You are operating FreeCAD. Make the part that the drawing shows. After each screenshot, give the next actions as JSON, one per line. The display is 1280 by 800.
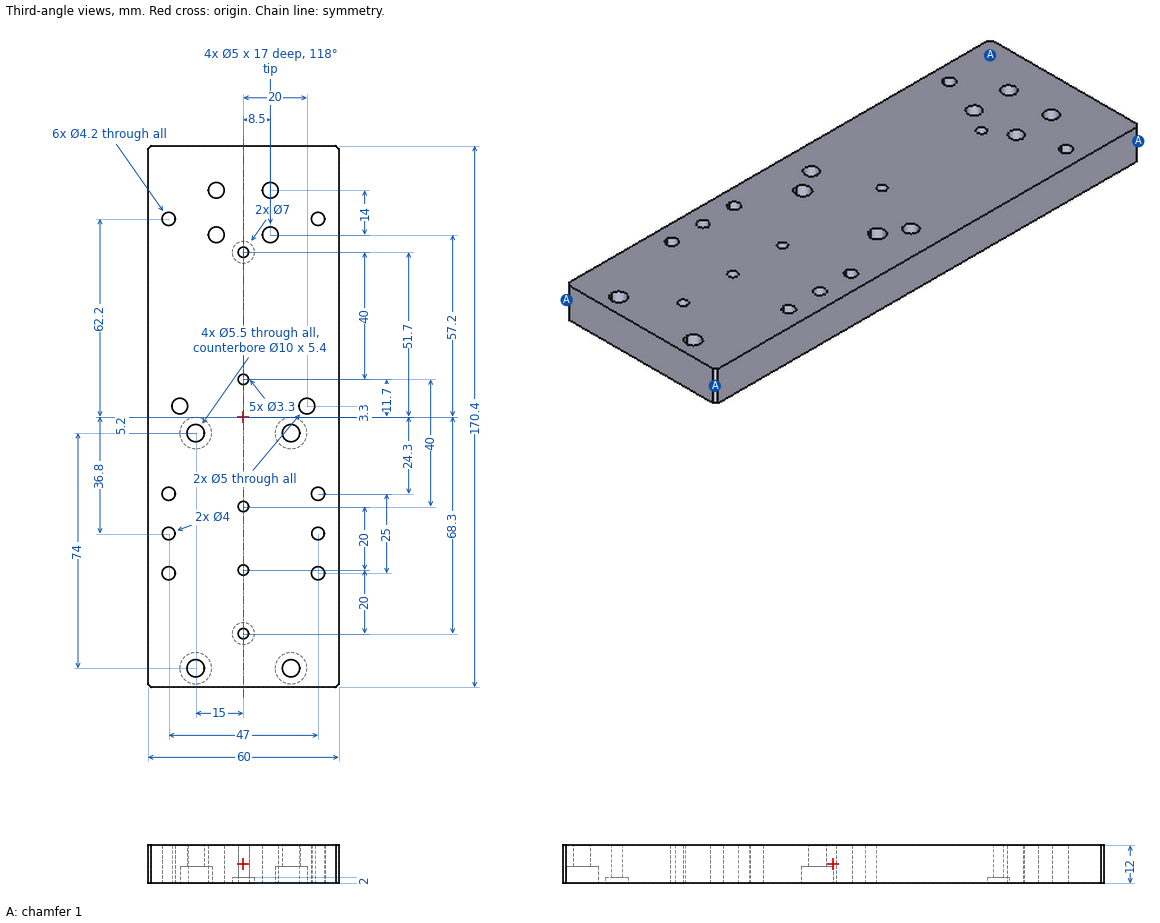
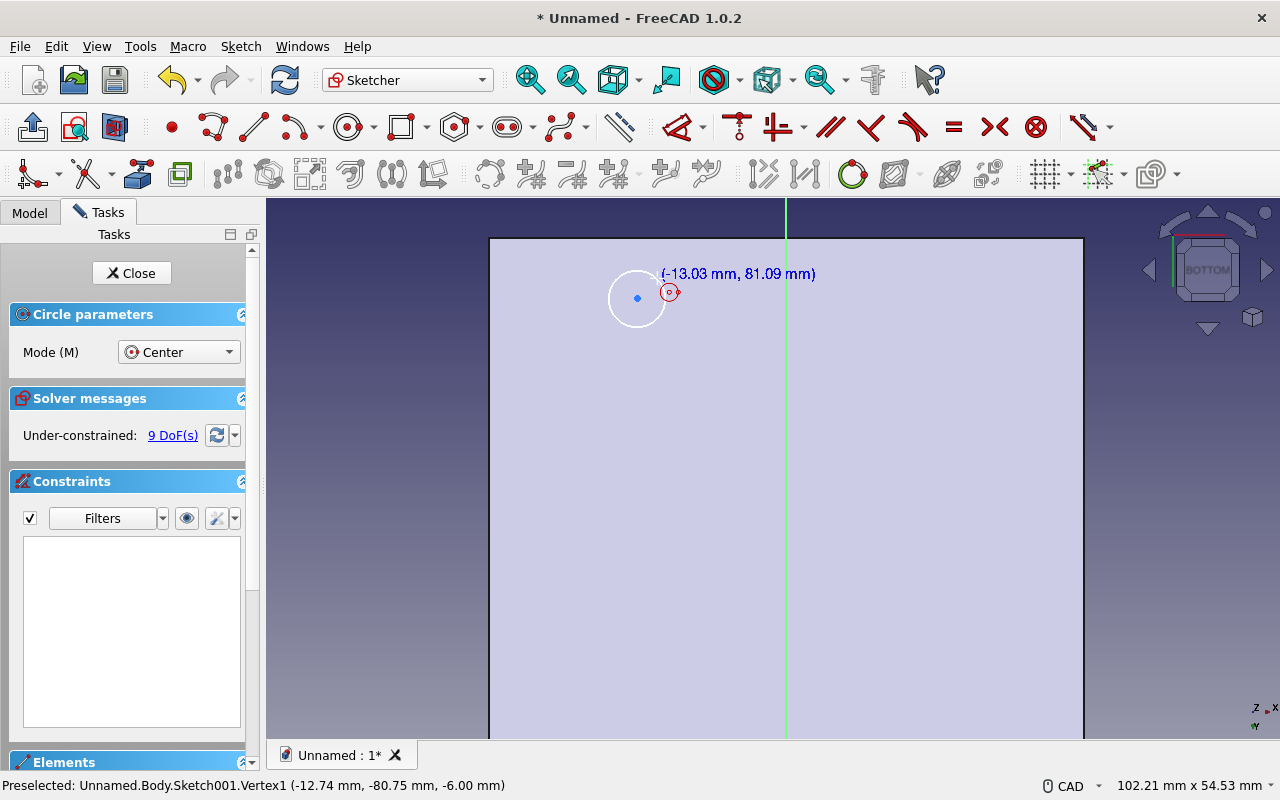
{"action": "left_click", "coordinate": [935, 298]}
{"action": "left_click", "coordinate": [954, 278]}
{"action": "key", "text": "Escape"}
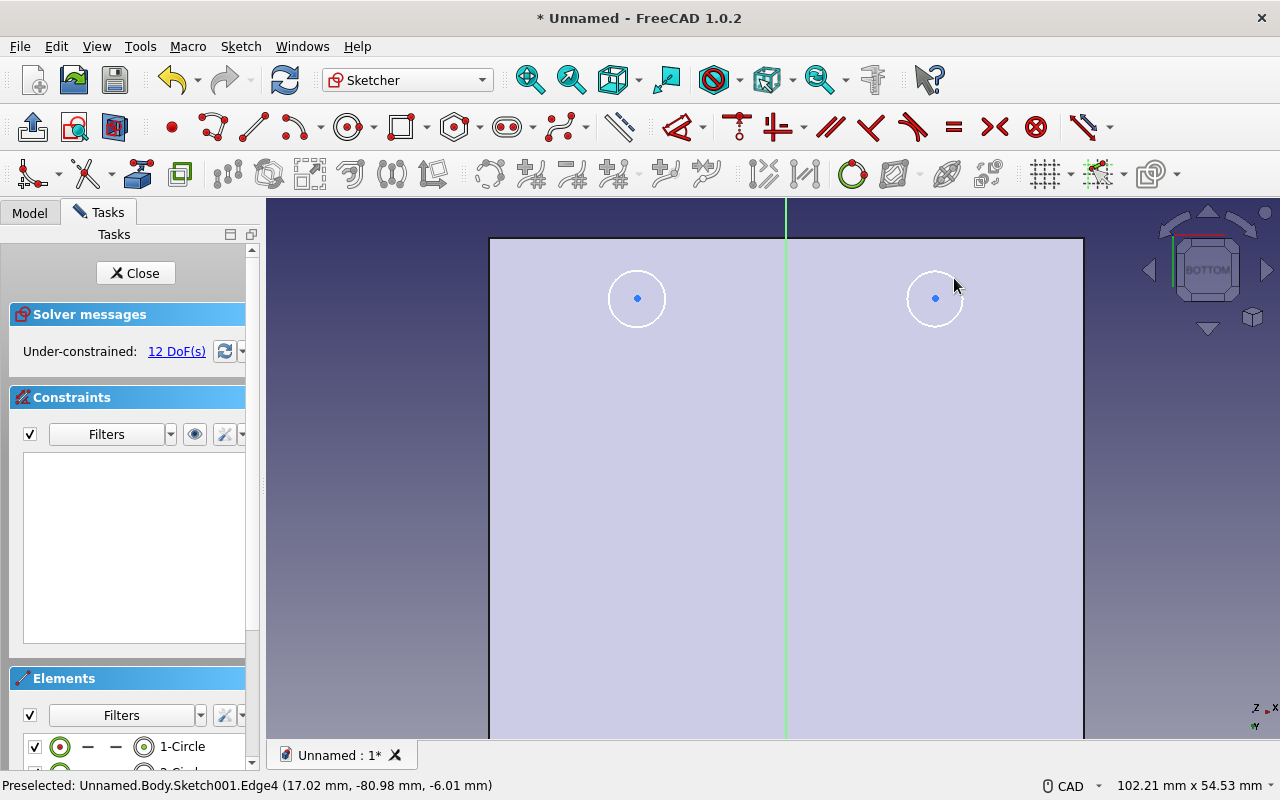
{"action": "scroll", "coordinate": [638, 298], "scroll_direction": "down", "scroll_amount": 4}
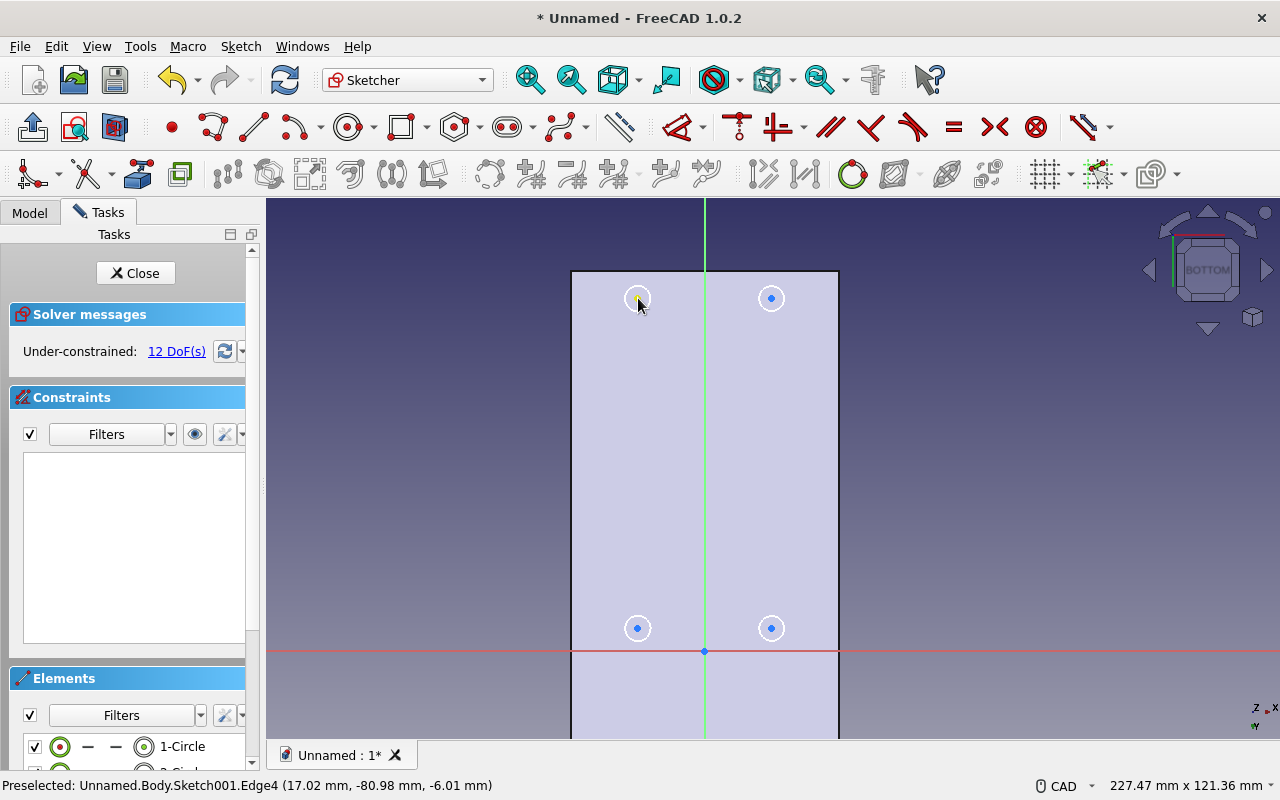
{"action": "left_click", "coordinate": [647, 619]}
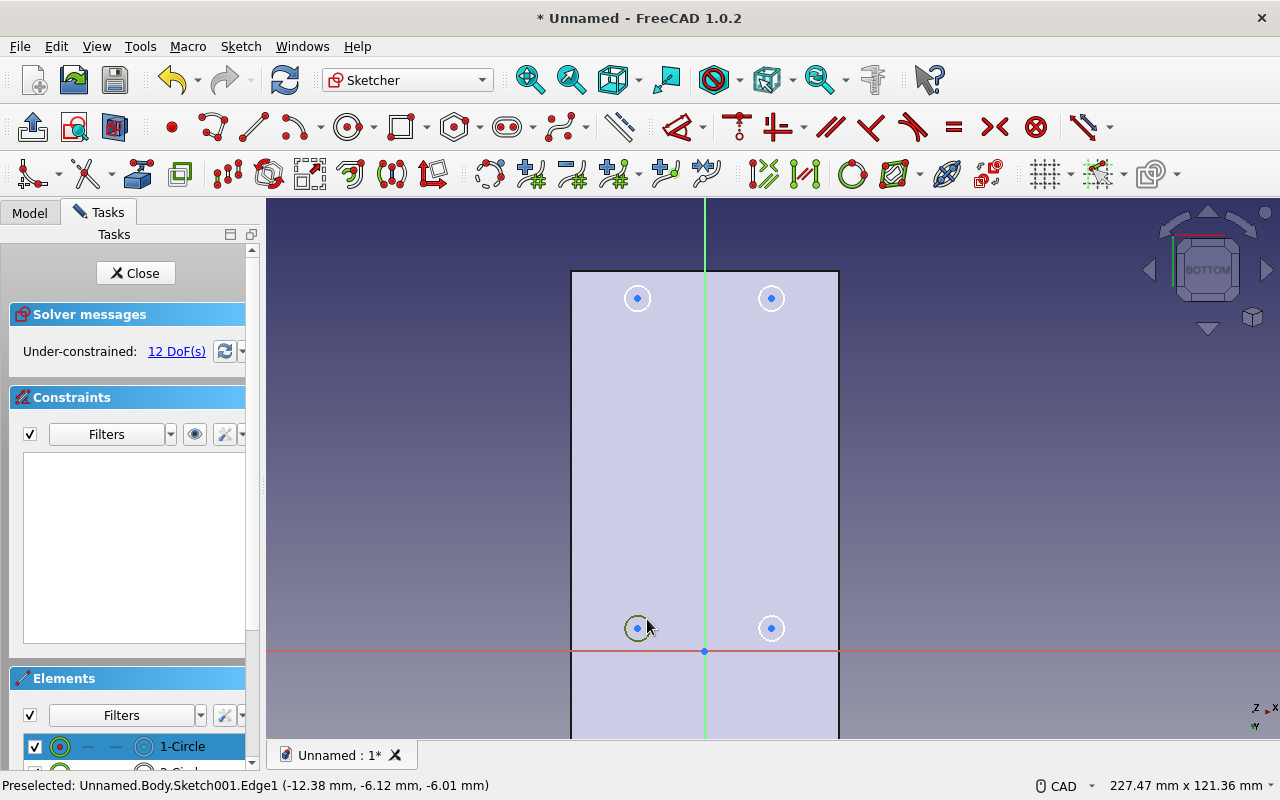
{"action": "left_click", "coordinate": [780, 620]}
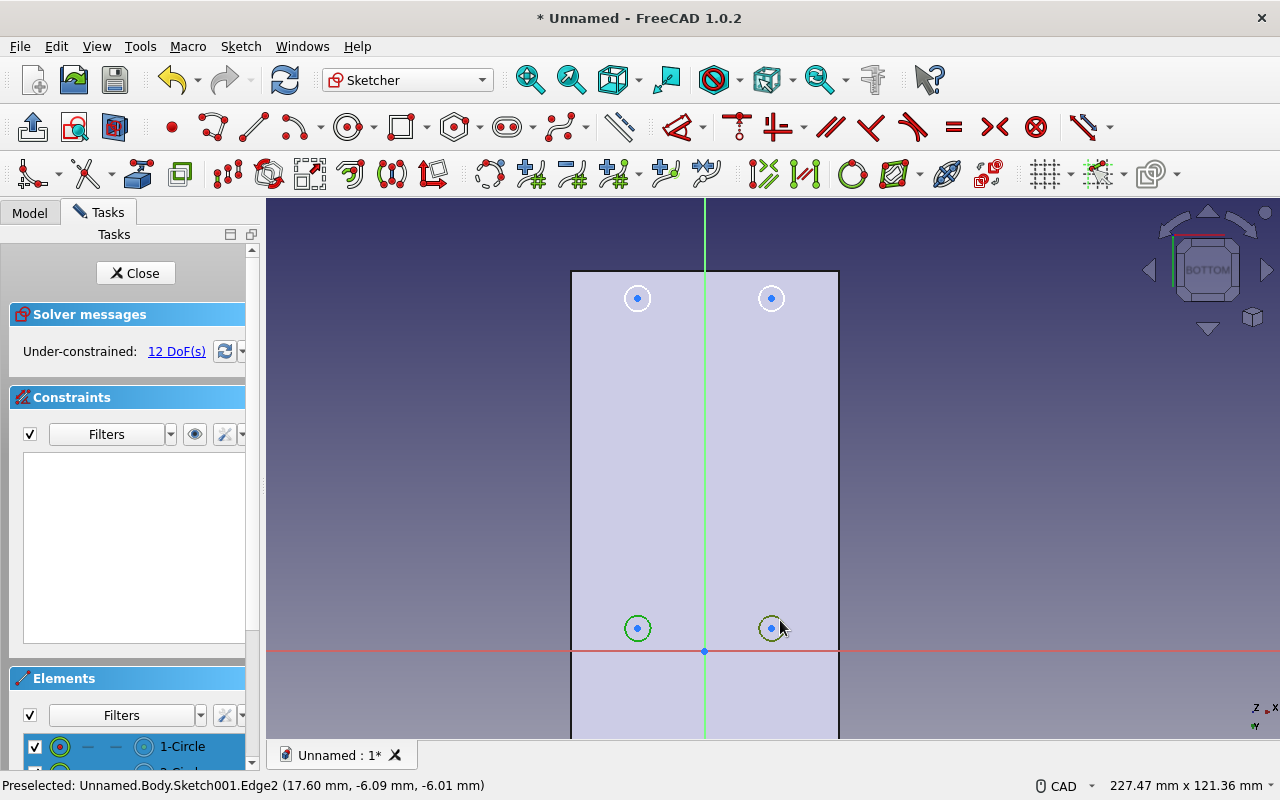
{"action": "left_click", "coordinate": [647, 290]}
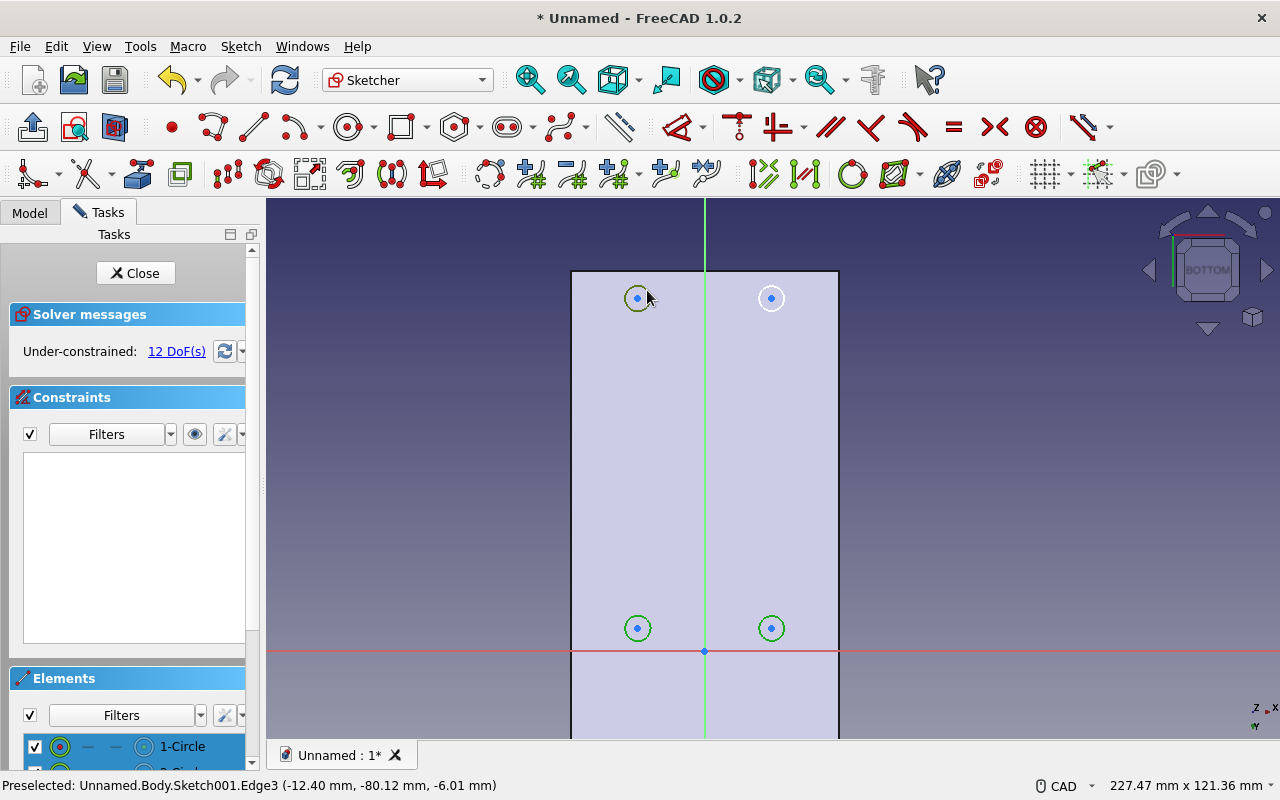
{"action": "left_click", "coordinate": [780, 290]}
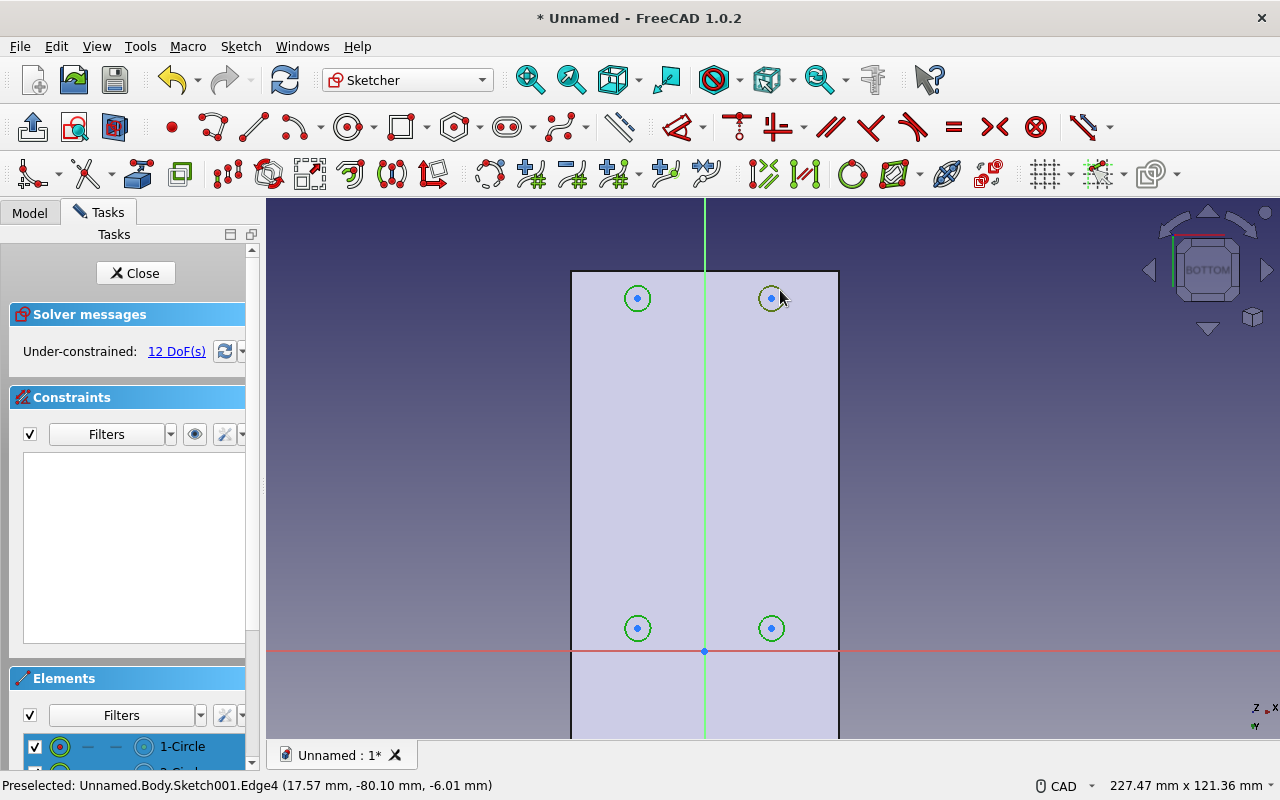
{"action": "left_click", "coordinate": [954, 128]}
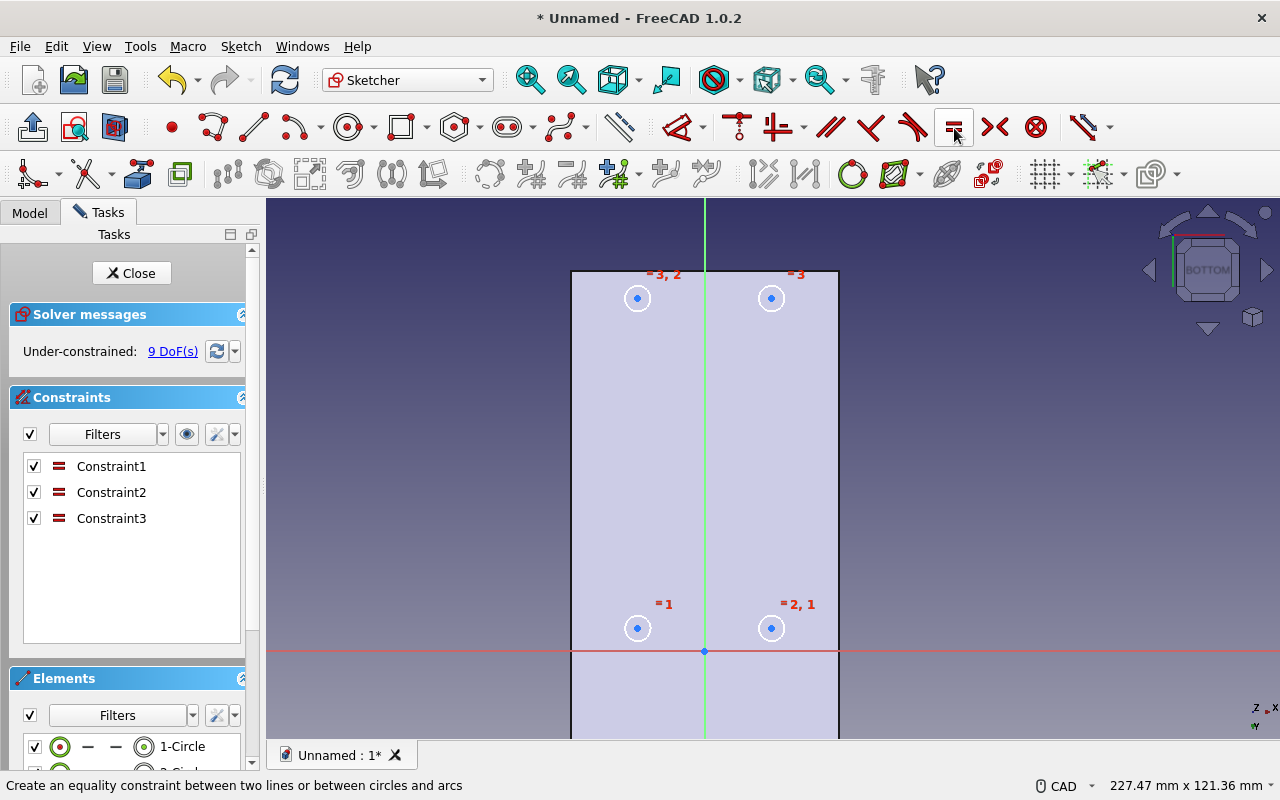
{"action": "left_click", "coordinate": [638, 628]}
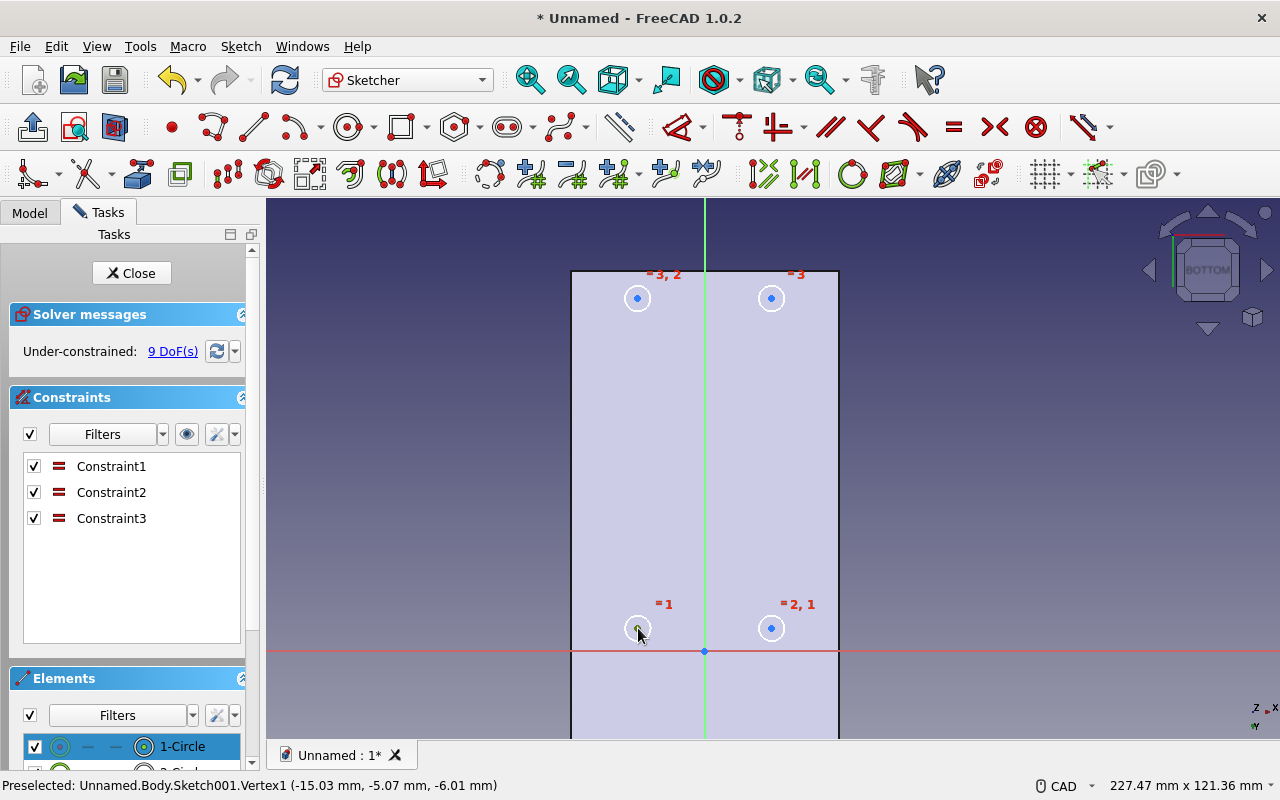
{"action": "left_click", "coordinate": [772, 628]}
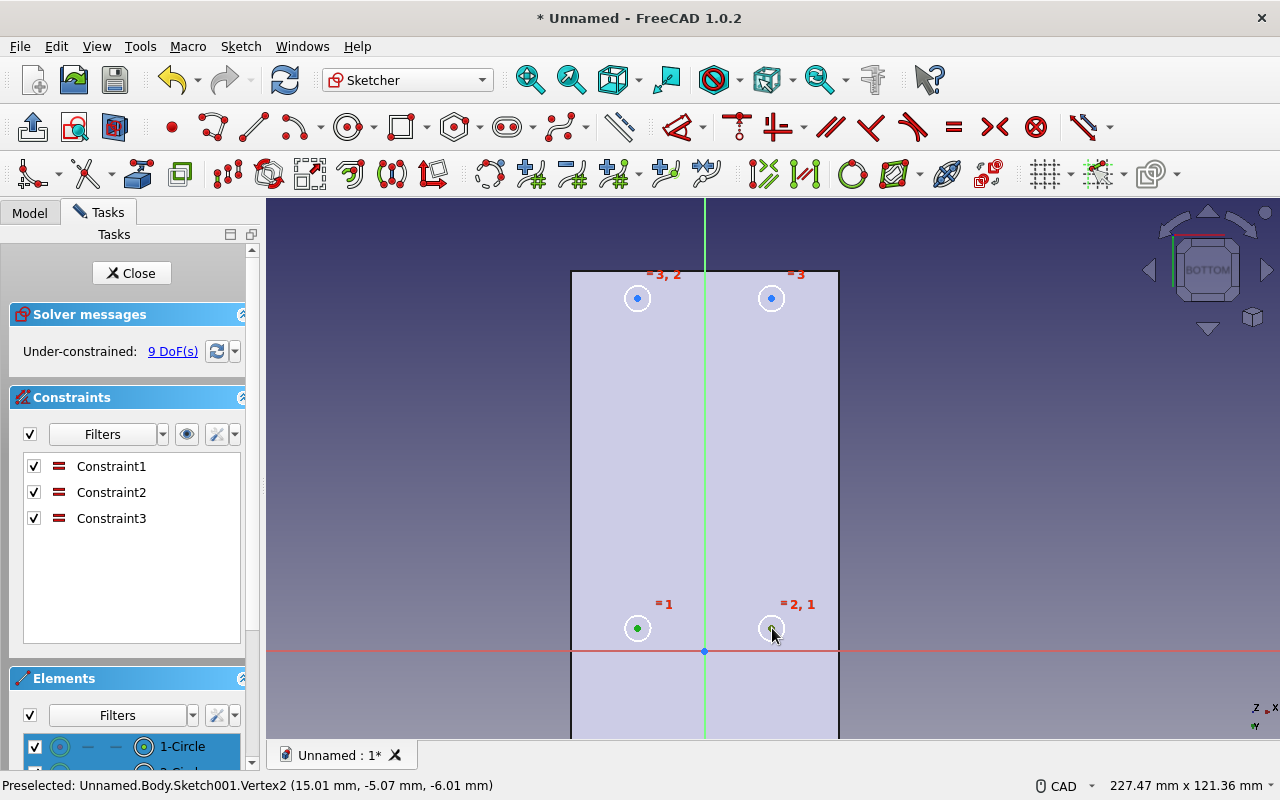
{"action": "left_click", "coordinate": [705, 607]}